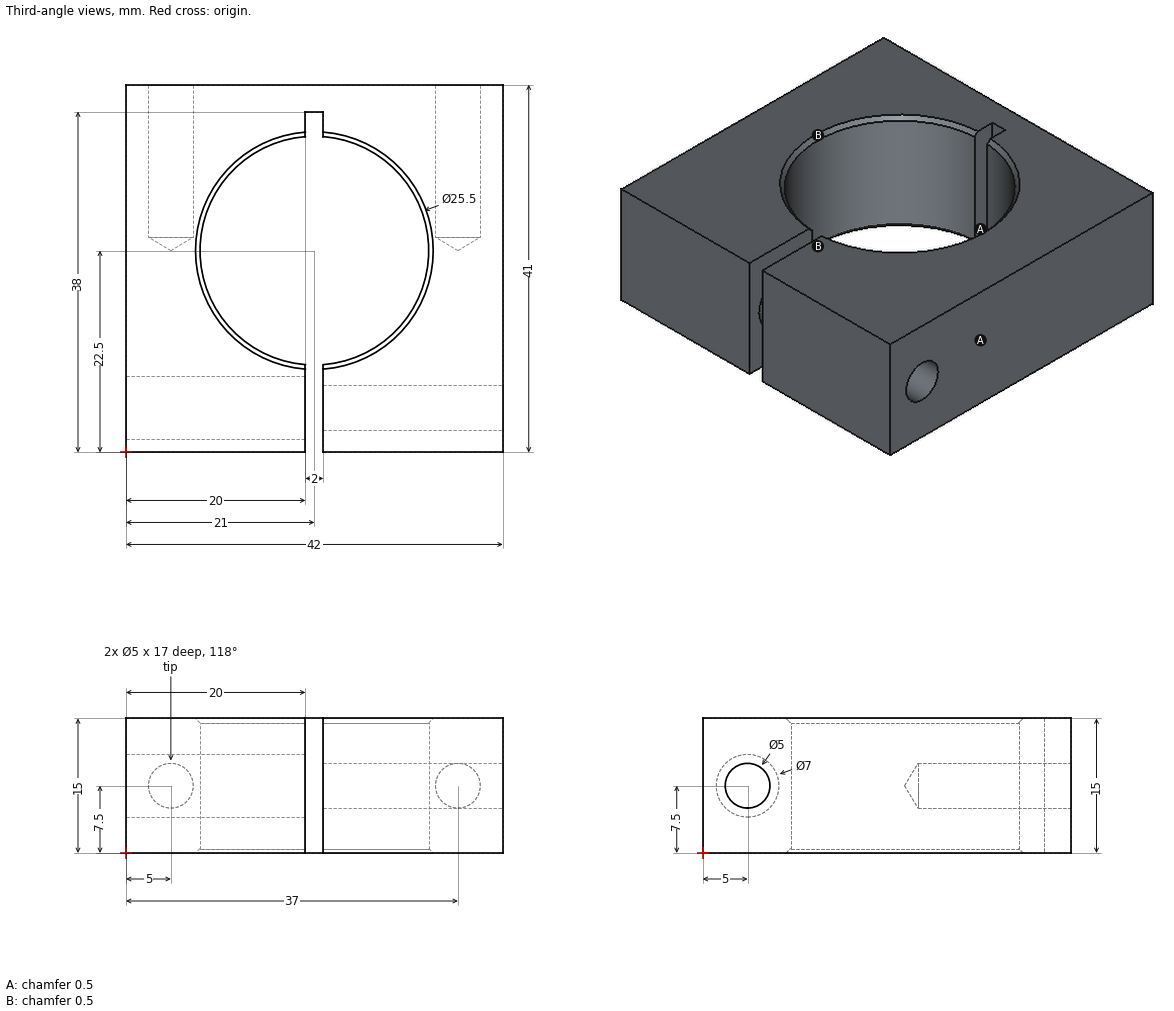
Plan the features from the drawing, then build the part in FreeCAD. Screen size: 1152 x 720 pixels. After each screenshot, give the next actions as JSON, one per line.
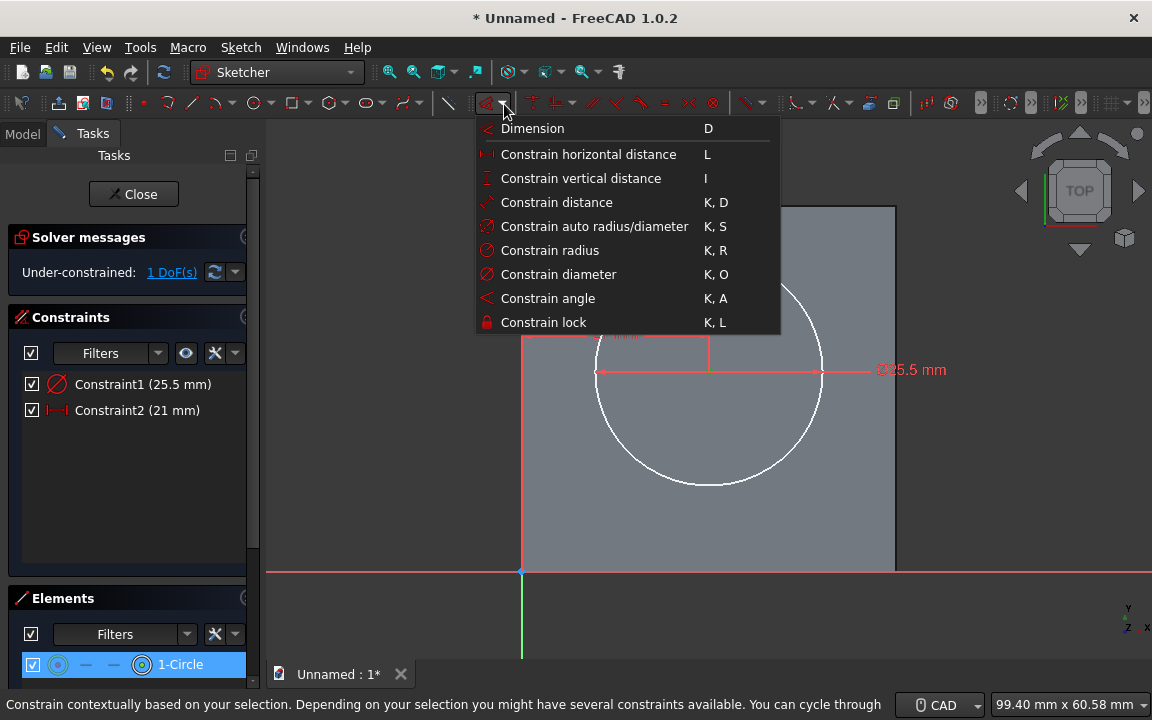
{"action": "left_click", "coordinate": [628, 178]}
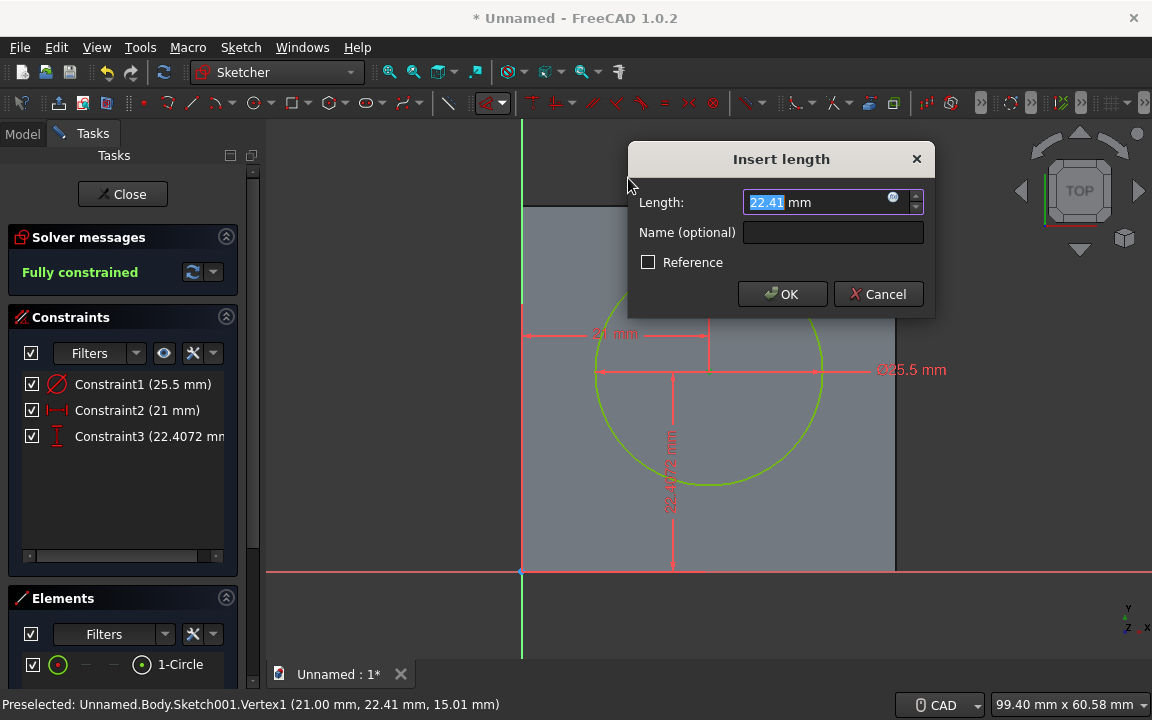
{"action": "type", "text": "22.5"}
{"action": "key", "text": "Return"}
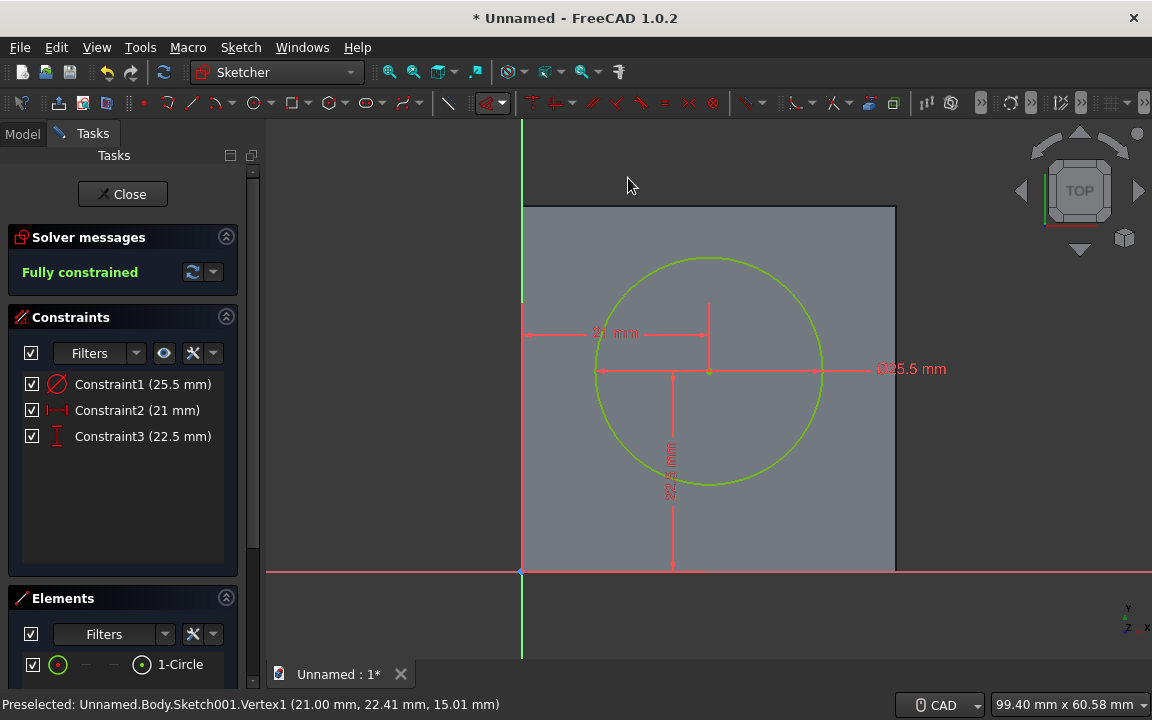
{"action": "left_click", "coordinate": [123, 194]}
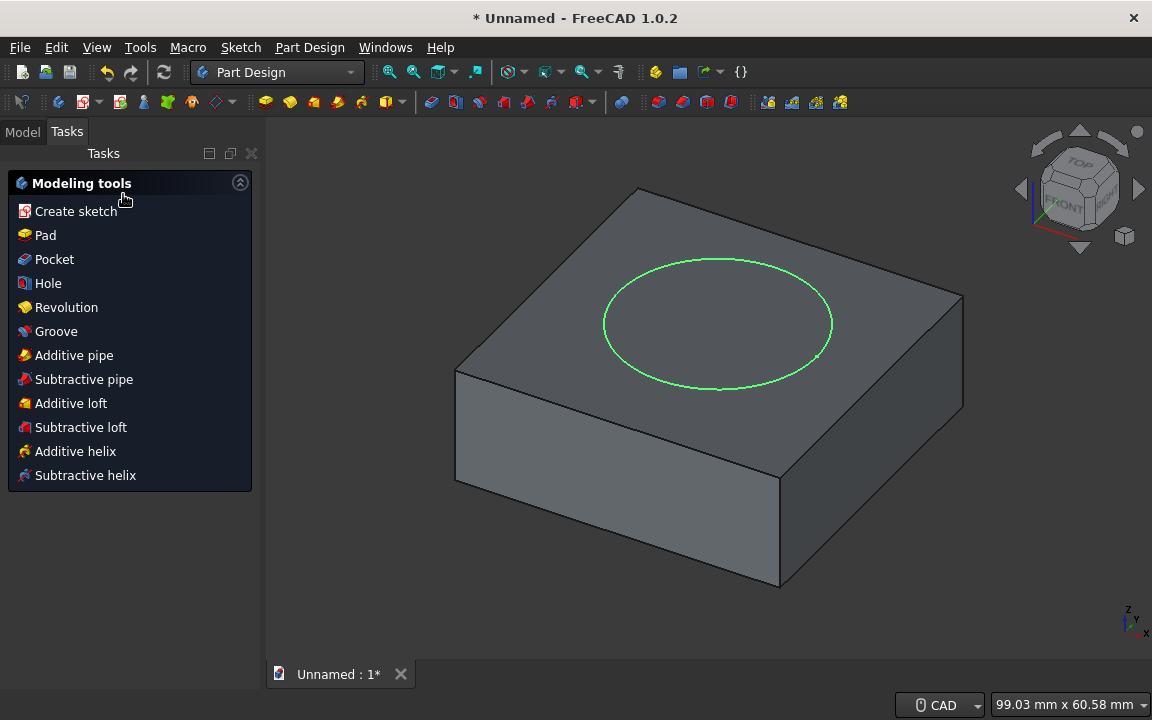
{"action": "left_click", "coordinate": [432, 102]}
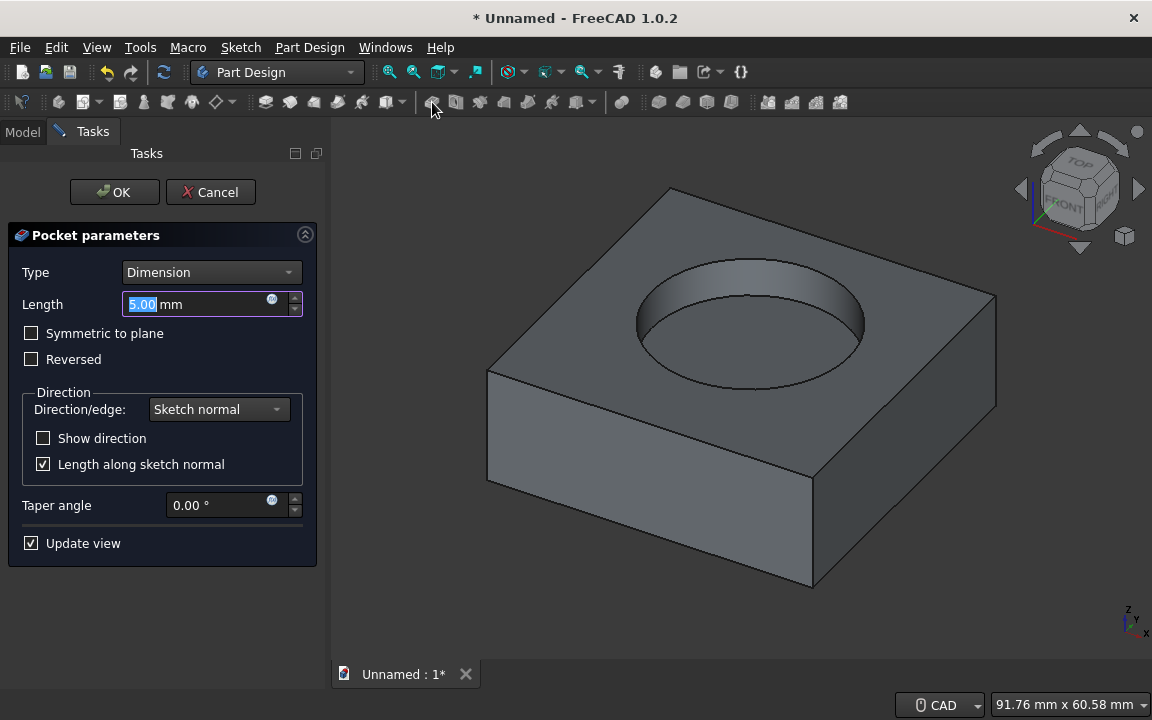
{"action": "type", "text": "15"}
{"action": "key", "text": "Tab"}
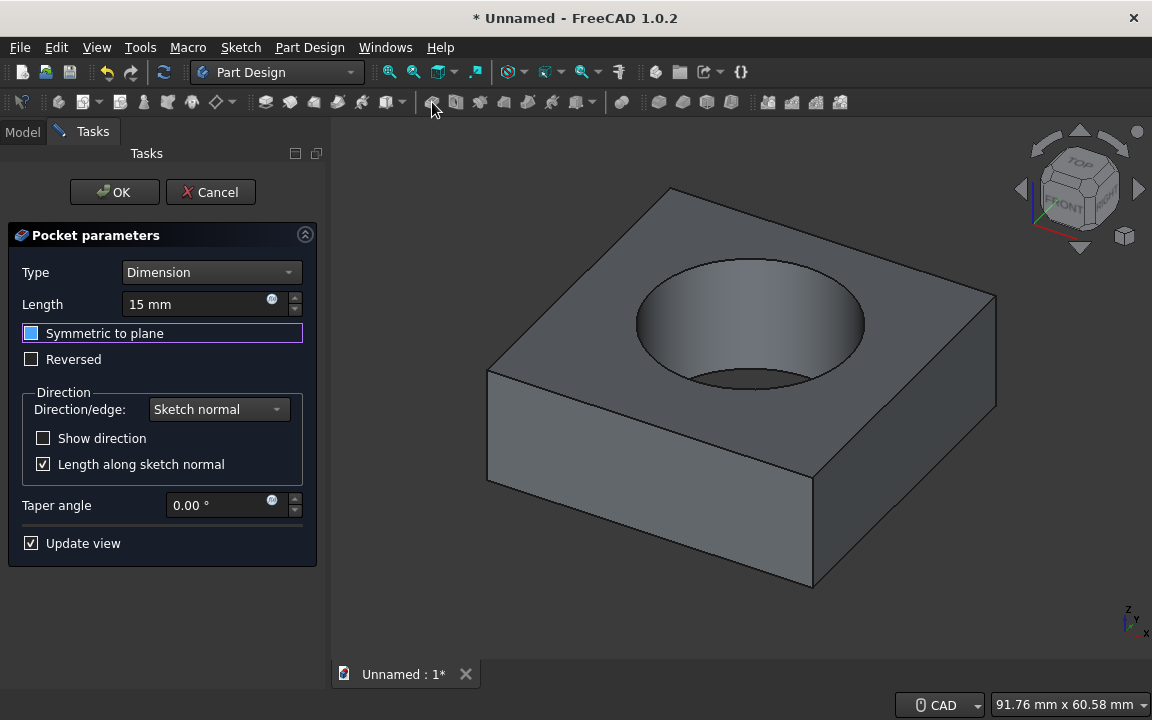
{"action": "left_click", "coordinate": [115, 192]}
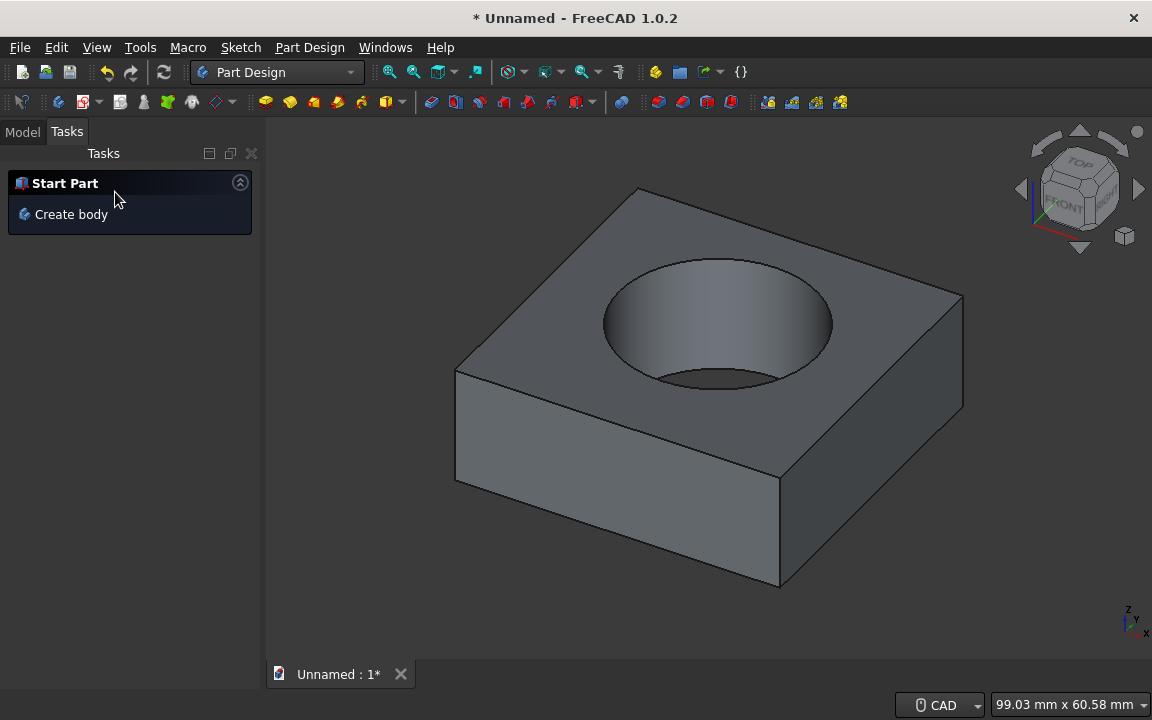
{"action": "left_click", "coordinate": [750, 415]}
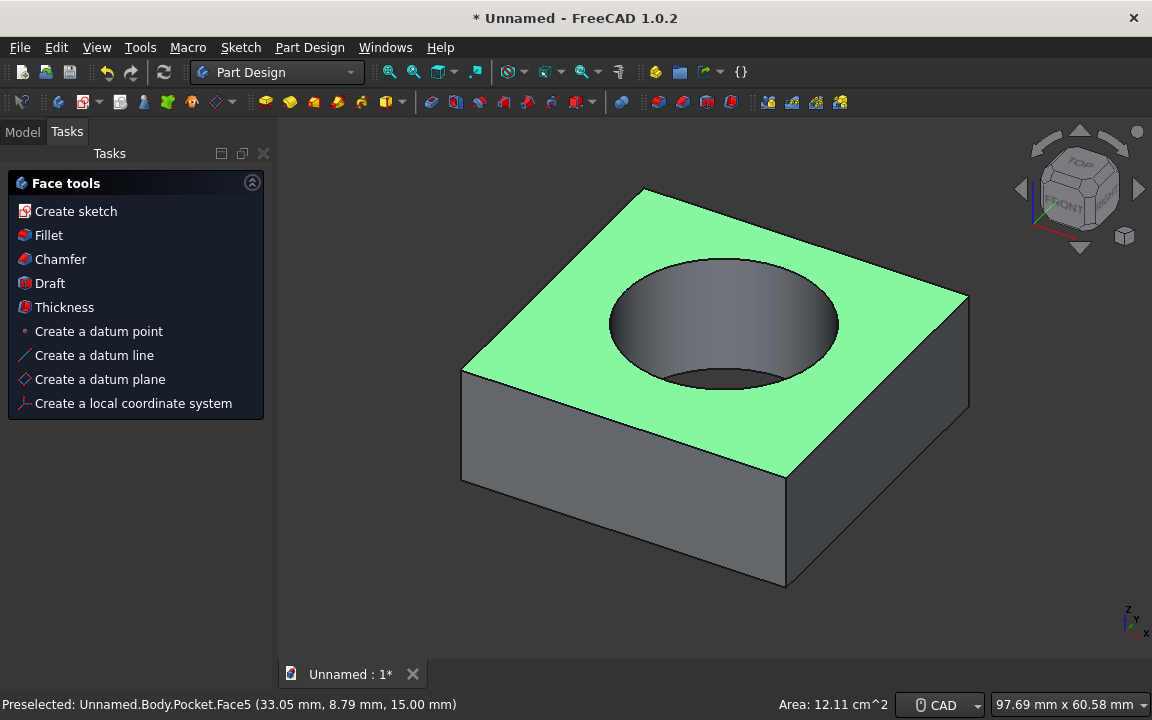
{"action": "left_click", "coordinate": [84, 102]}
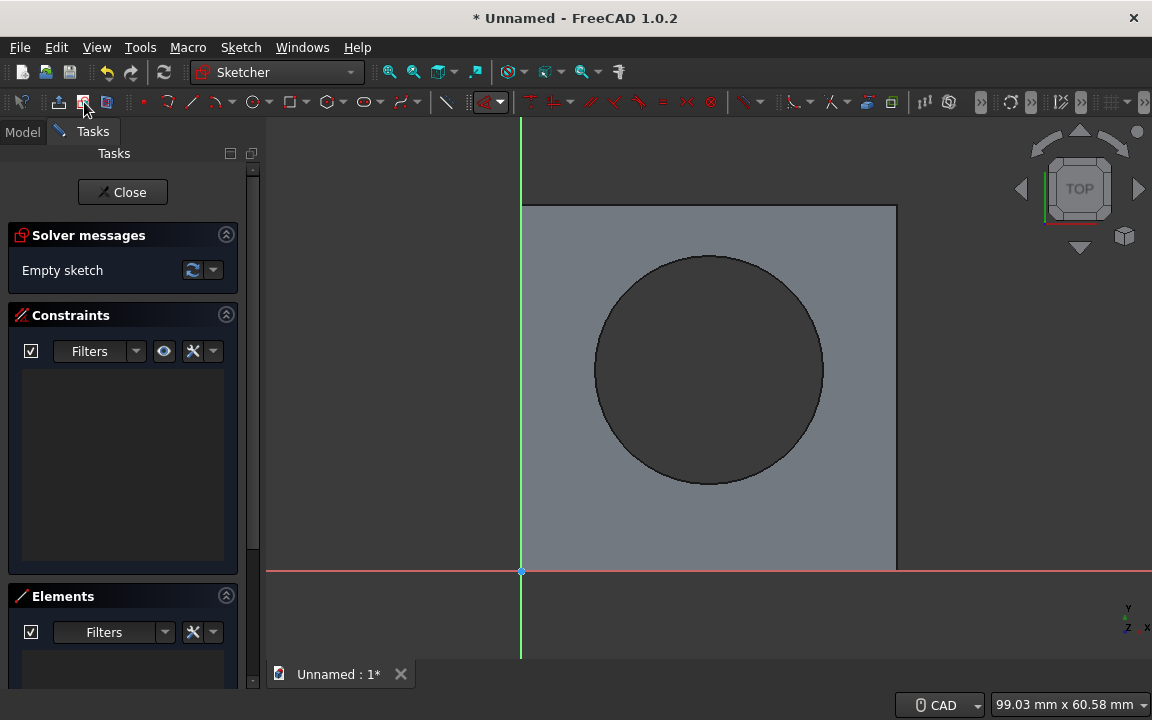
{"action": "left_click", "coordinate": [290, 102]}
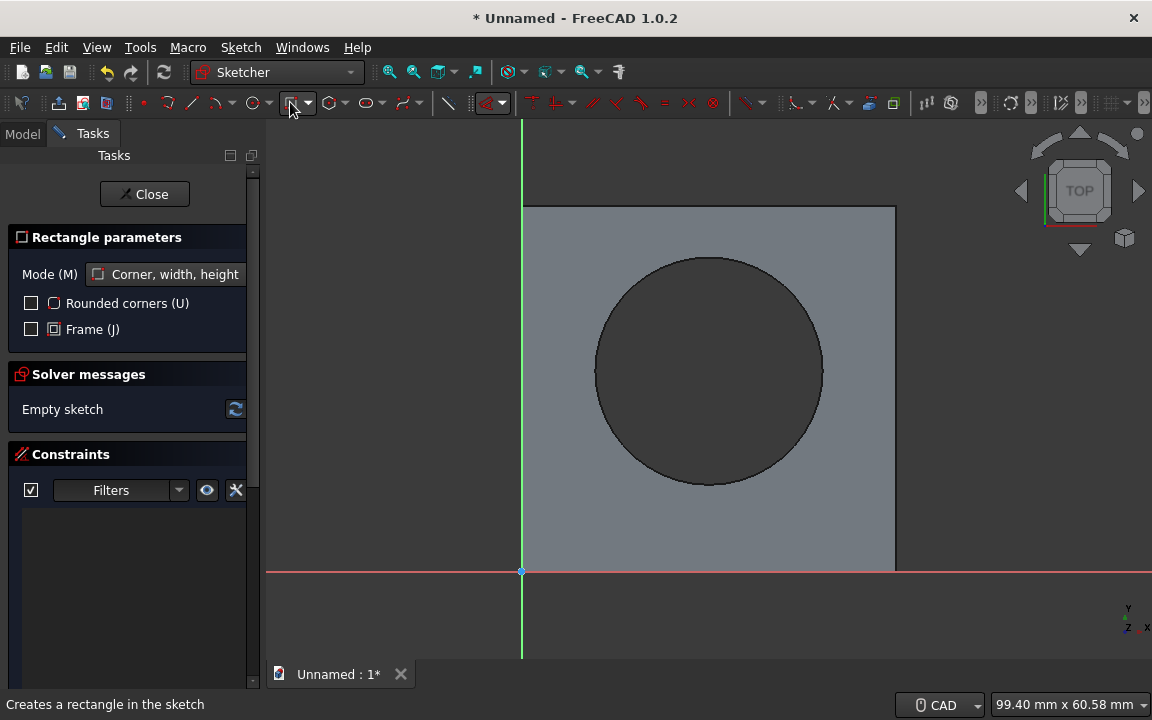
{"action": "left_click", "coordinate": [700, 233]}
{"action": "left_click", "coordinate": [718, 572]}
{"action": "key", "text": "Escape"}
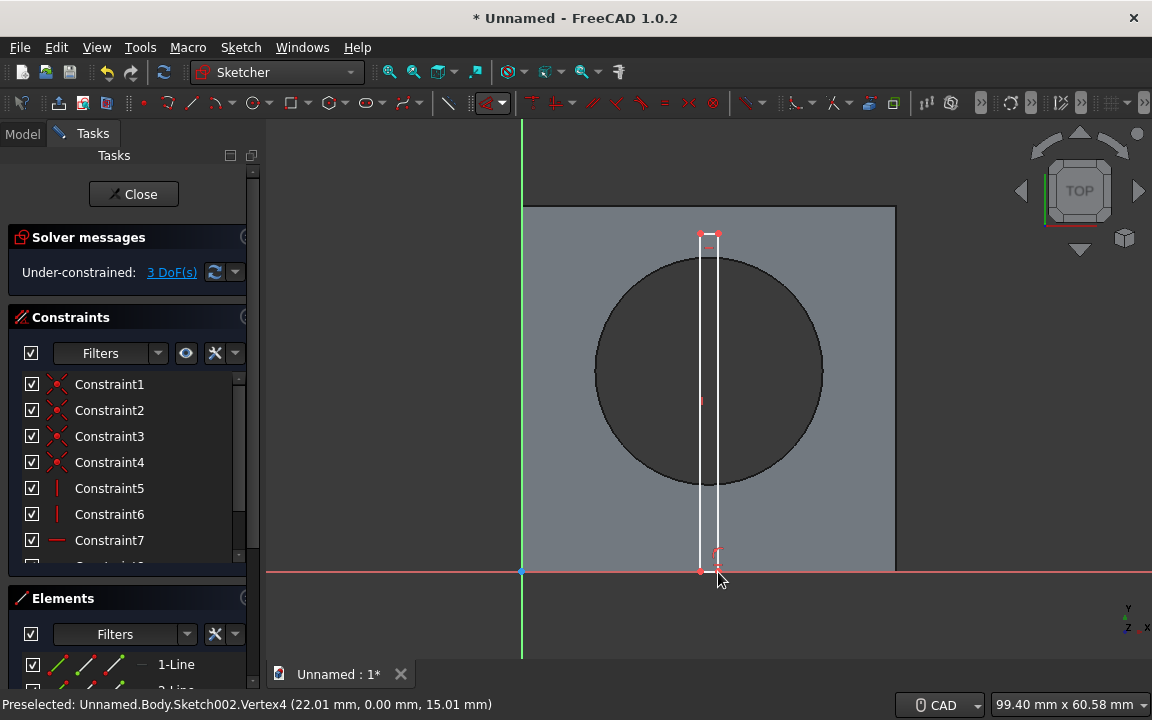
{"action": "scroll", "coordinate": [709, 572], "scroll_direction": "up", "scroll_amount": 5}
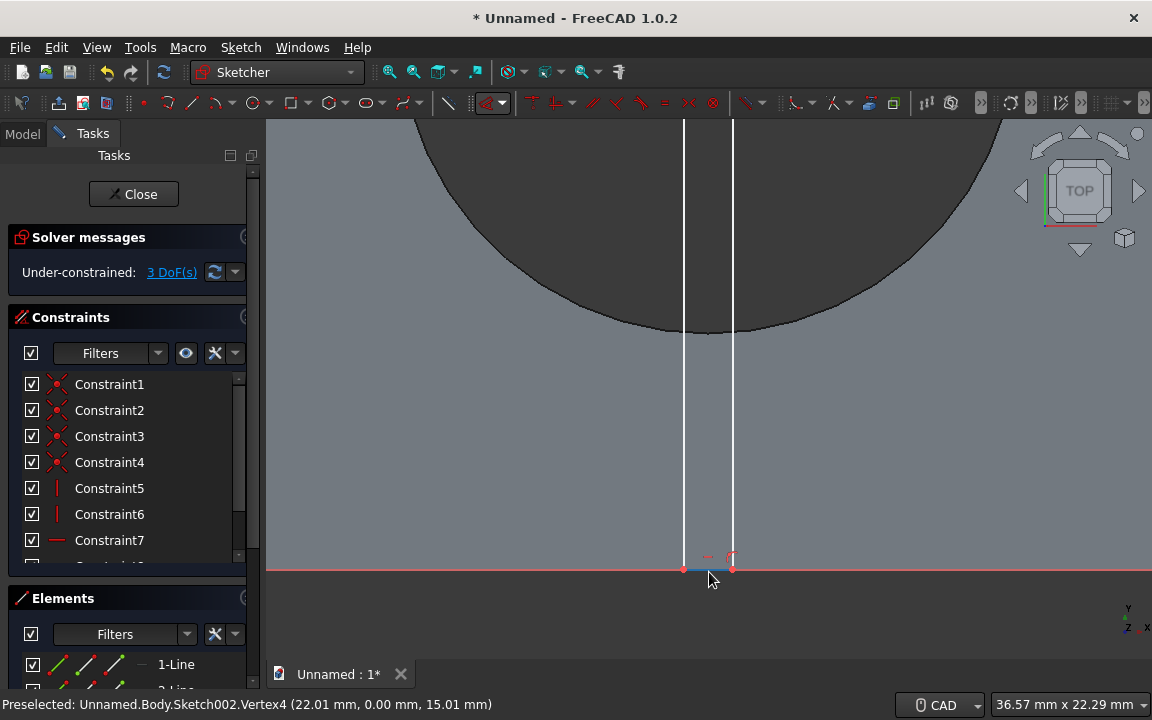
{"action": "left_click", "coordinate": [708, 570]}